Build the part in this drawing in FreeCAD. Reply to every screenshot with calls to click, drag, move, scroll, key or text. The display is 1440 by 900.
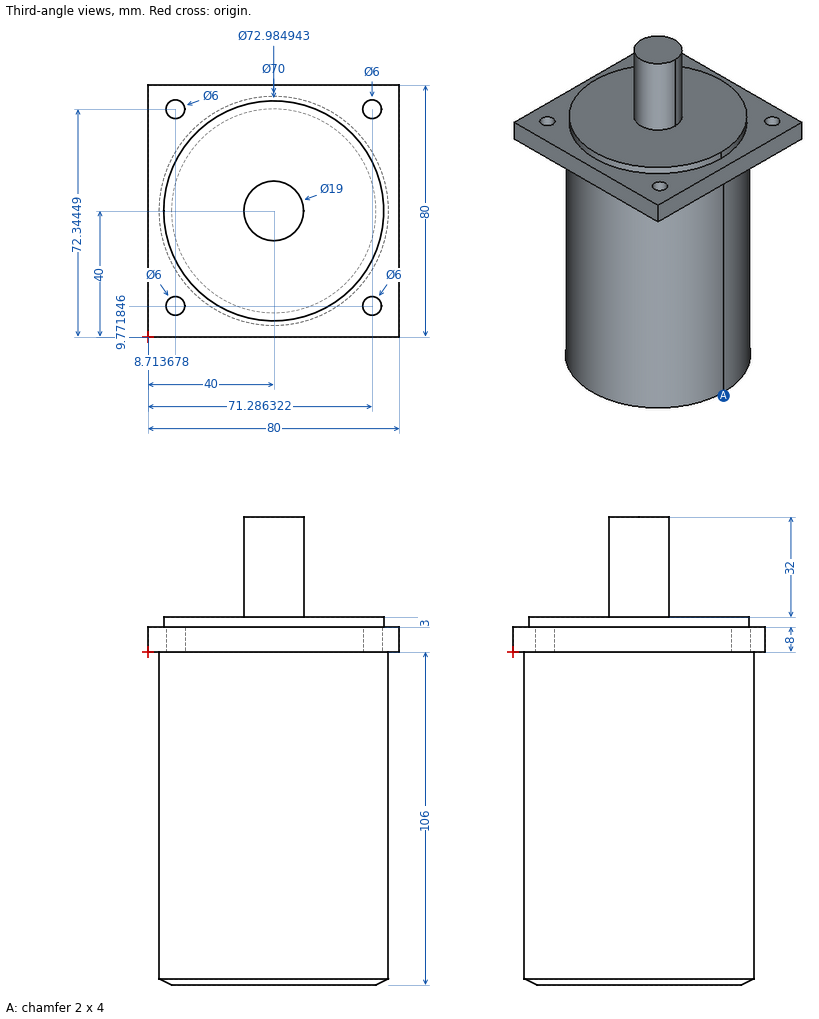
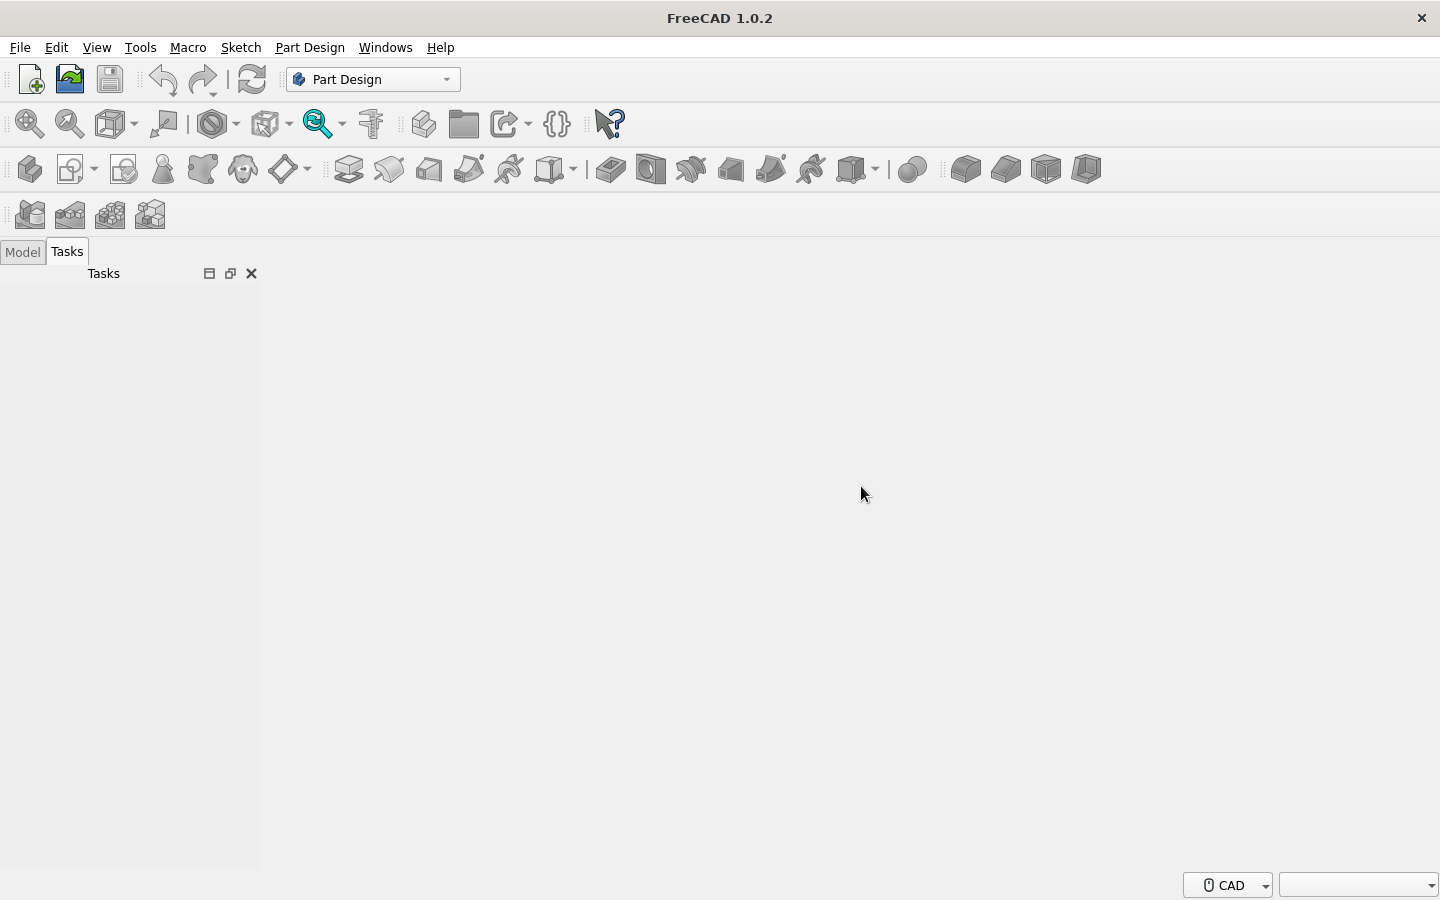
click(30, 80)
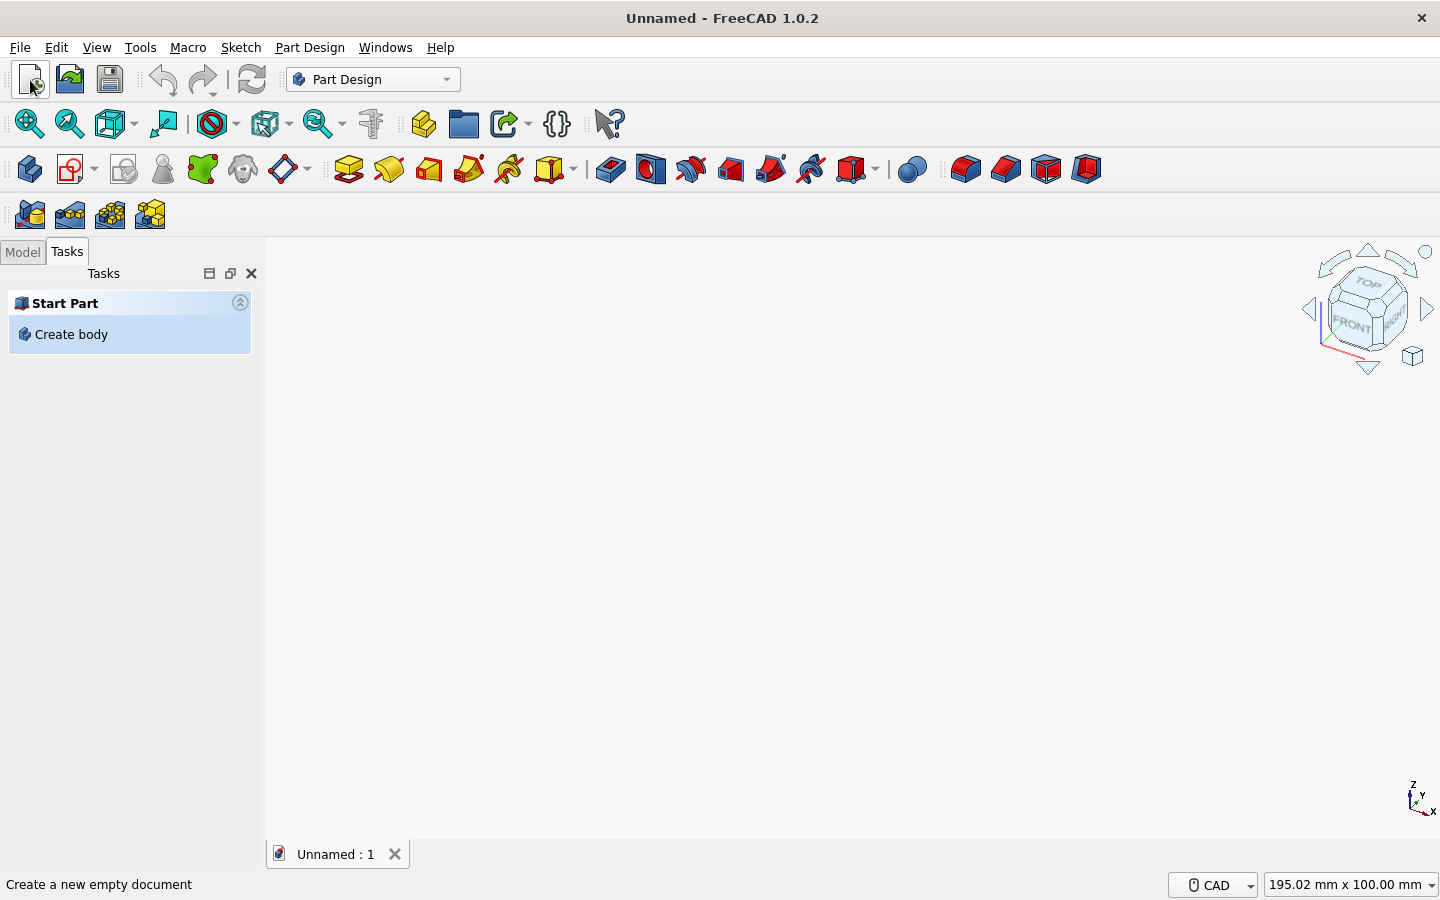
click(70, 170)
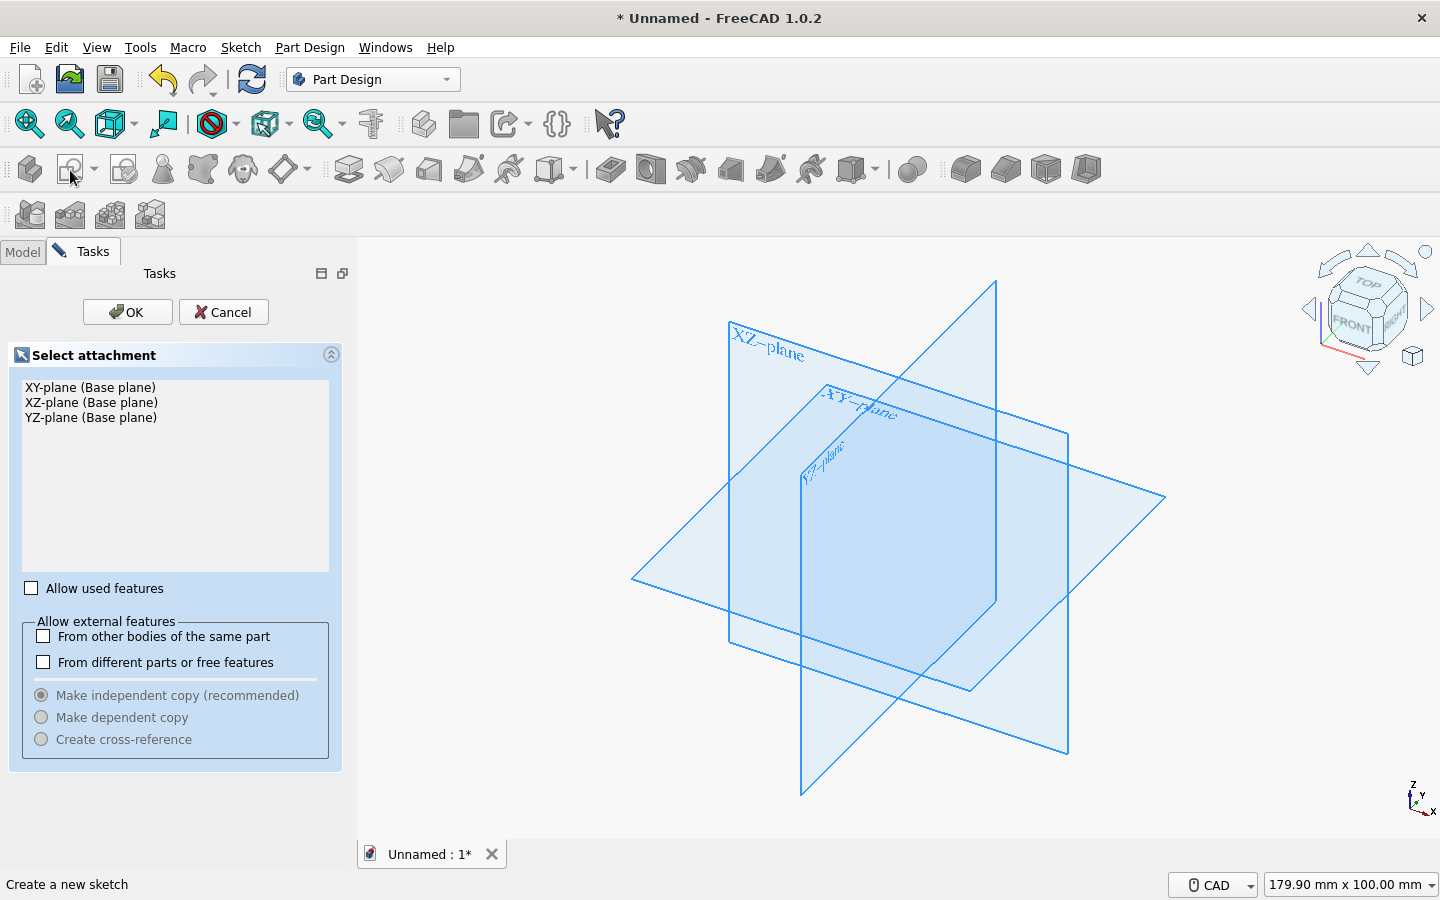
click(82, 388)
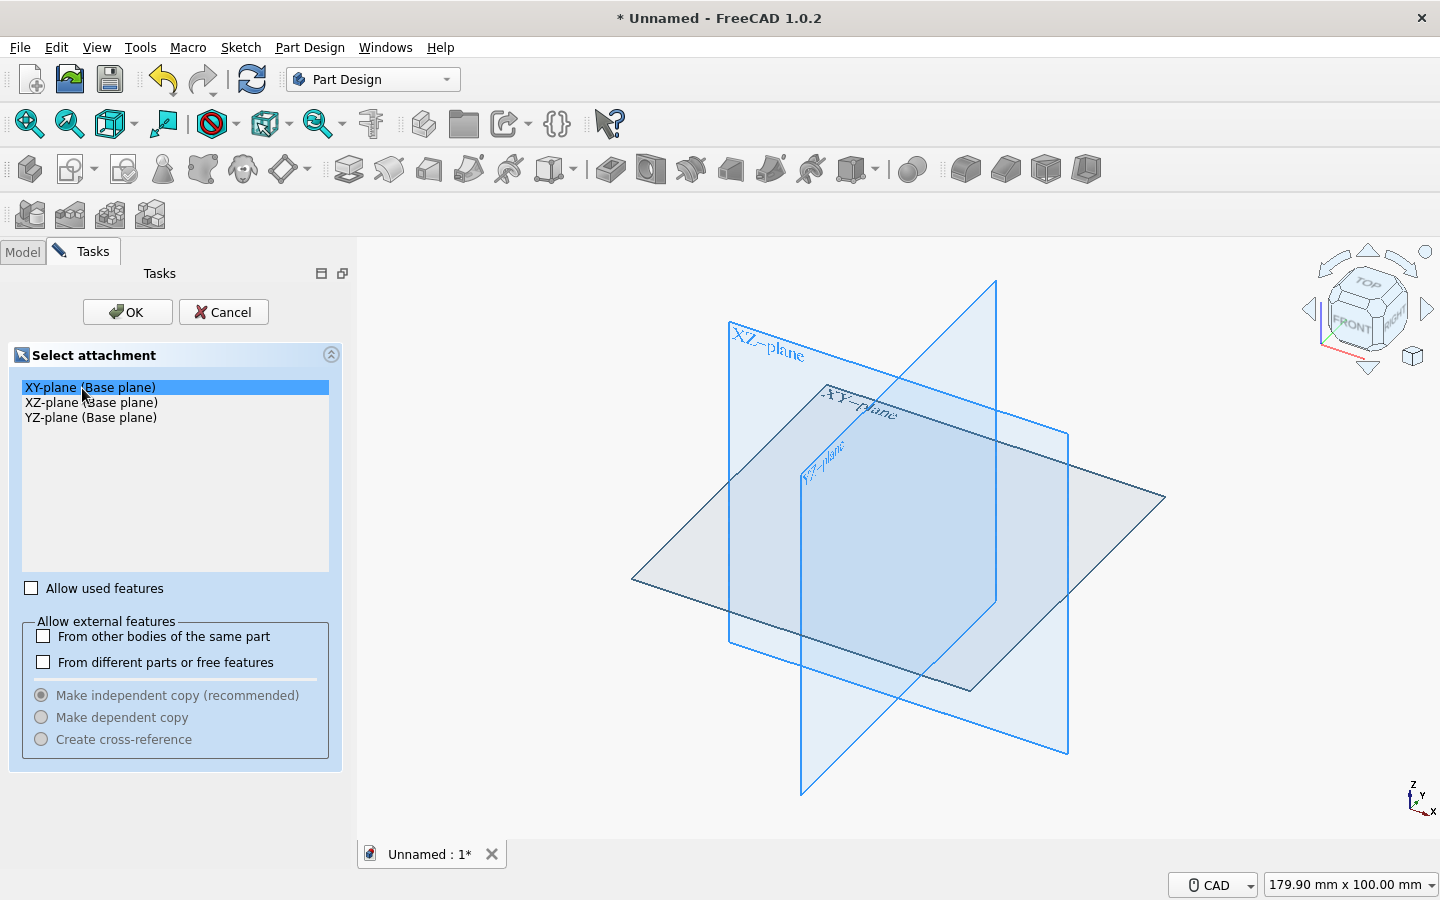
click(128, 312)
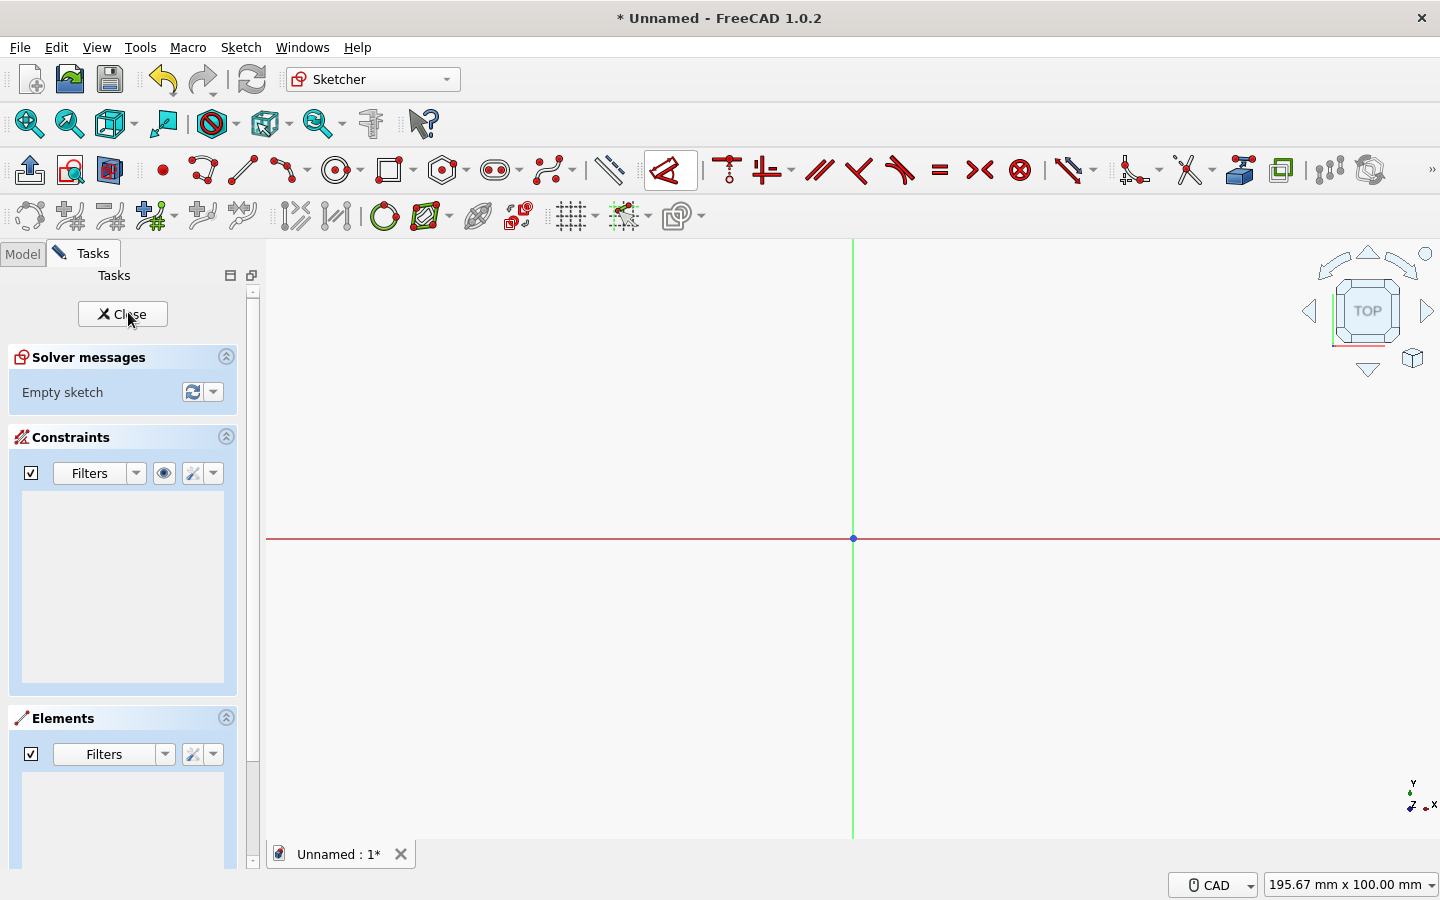
scroll(294, 811, down, 2)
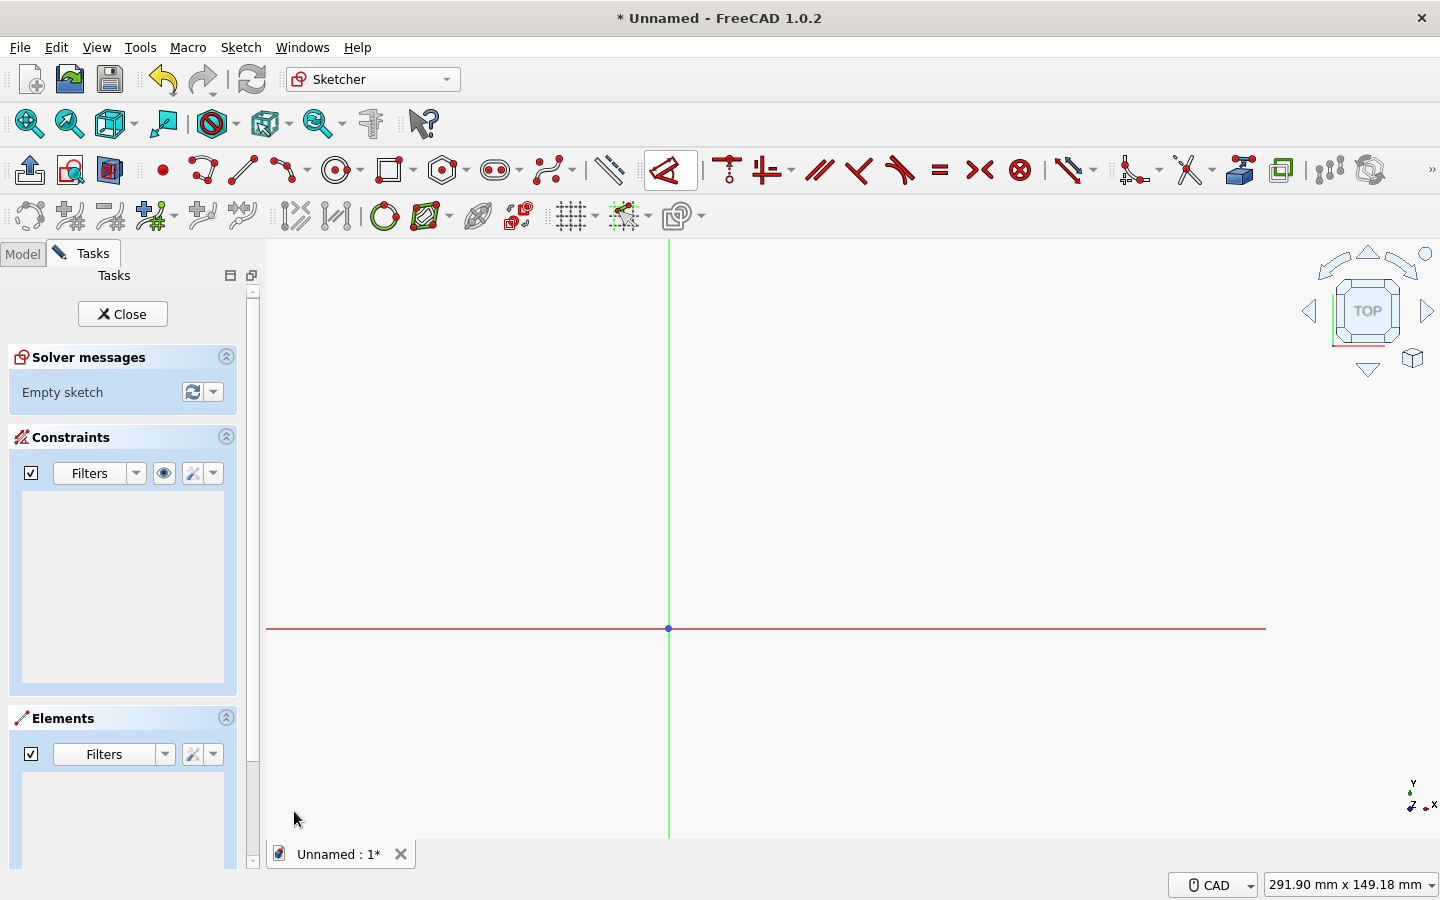
click(390, 170)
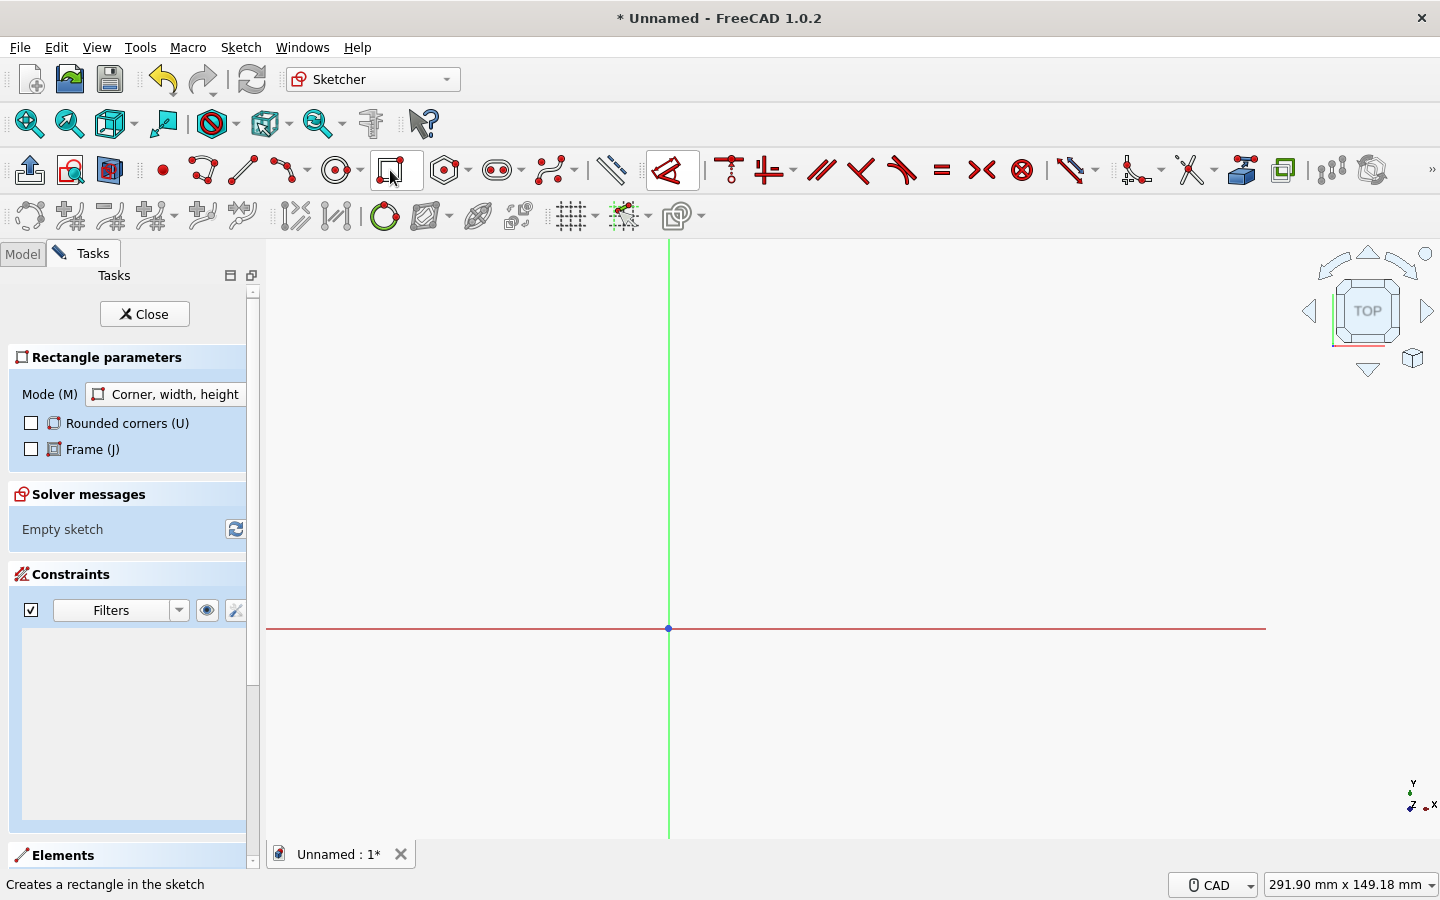
click(669, 629)
move(990, 307)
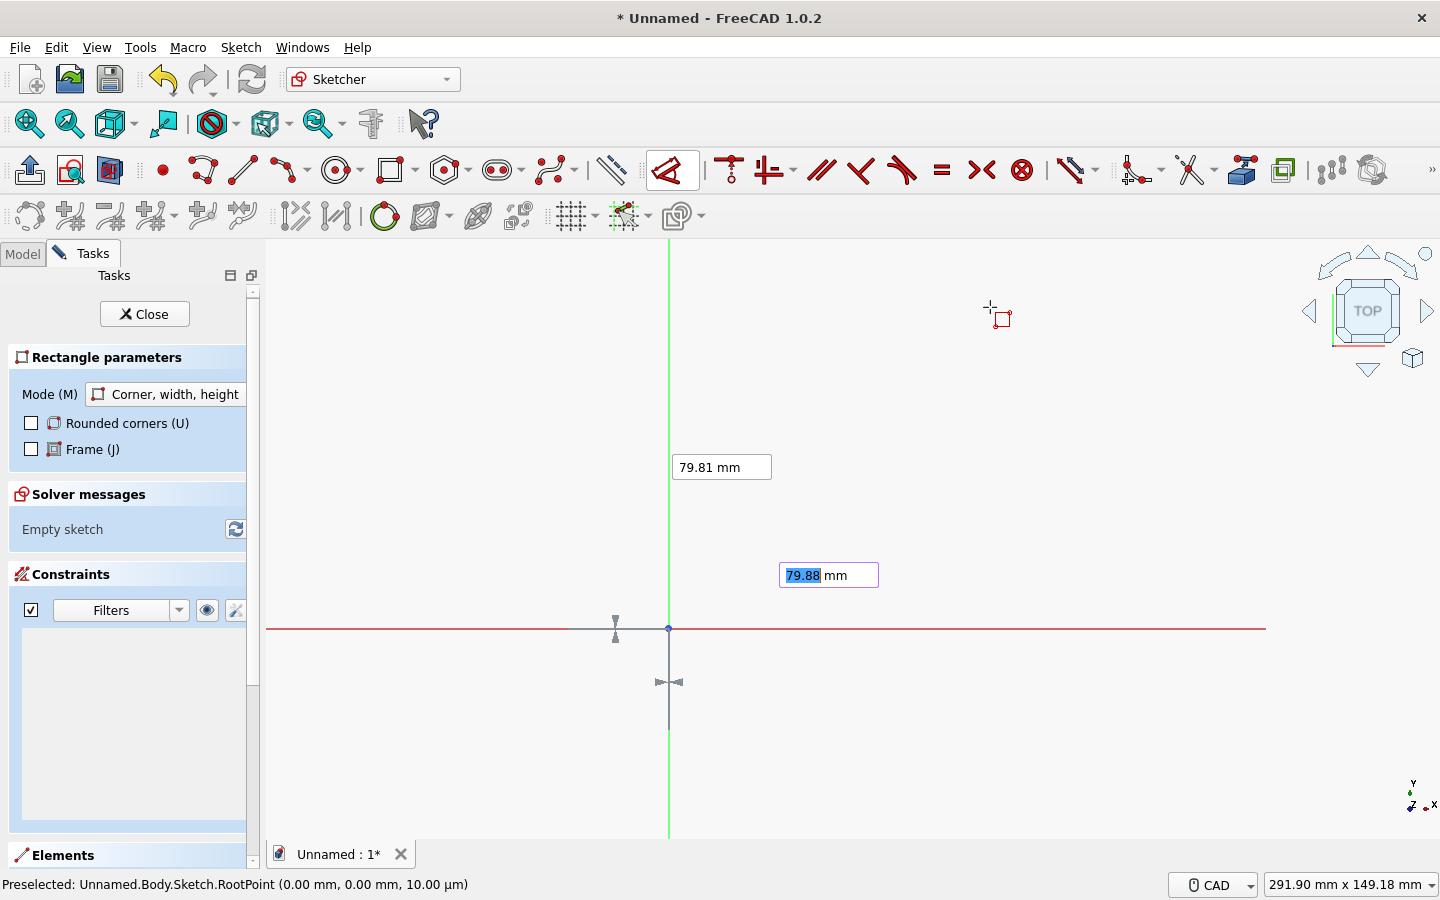
text(80)
key(Tab)
text(80)
key(Return)
key(Escape)